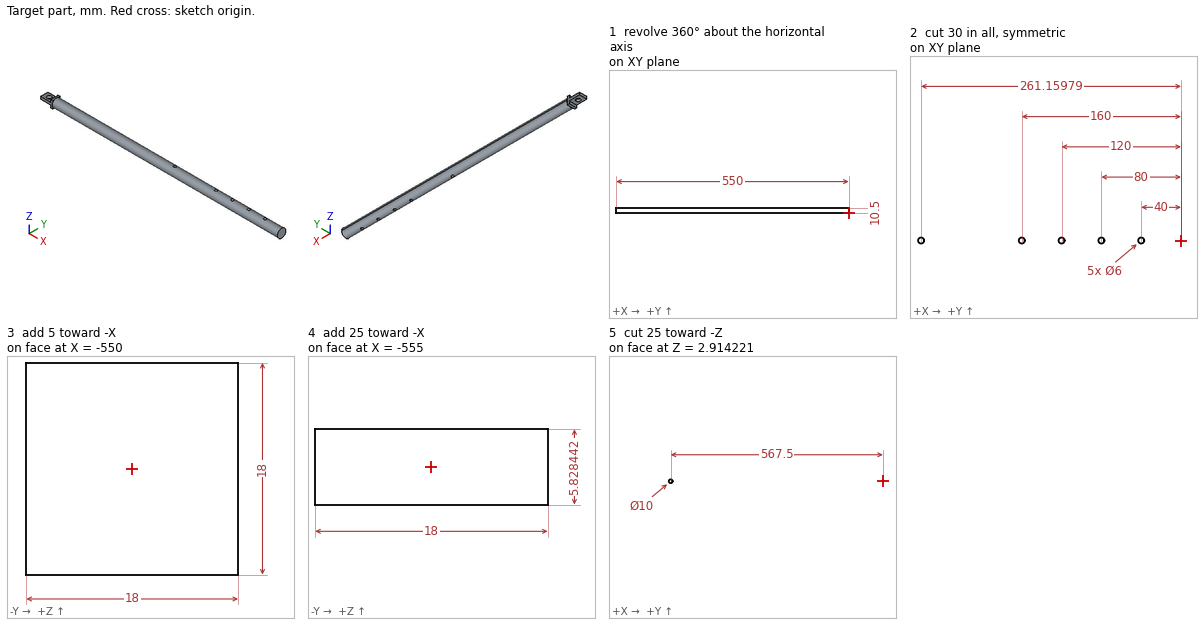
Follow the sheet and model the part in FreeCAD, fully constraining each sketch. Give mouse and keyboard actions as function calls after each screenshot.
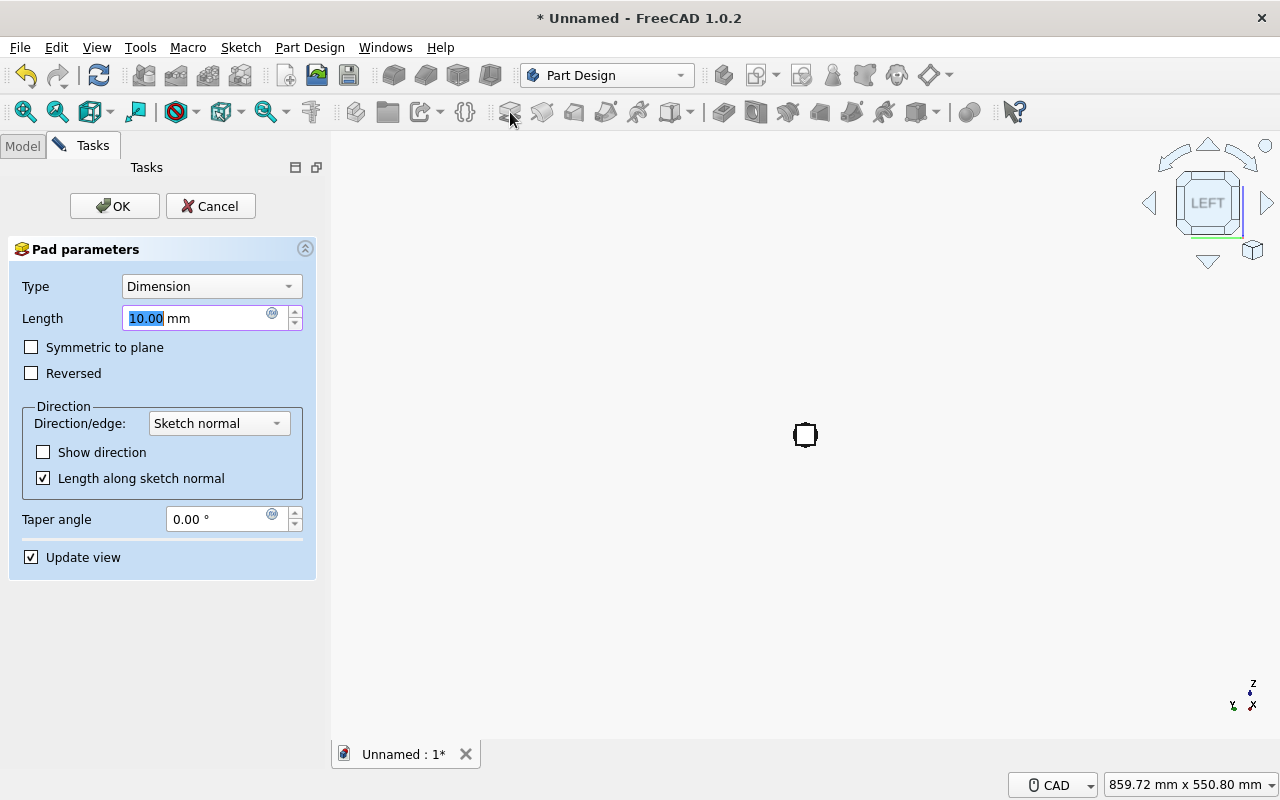
text(5)
key(Tab)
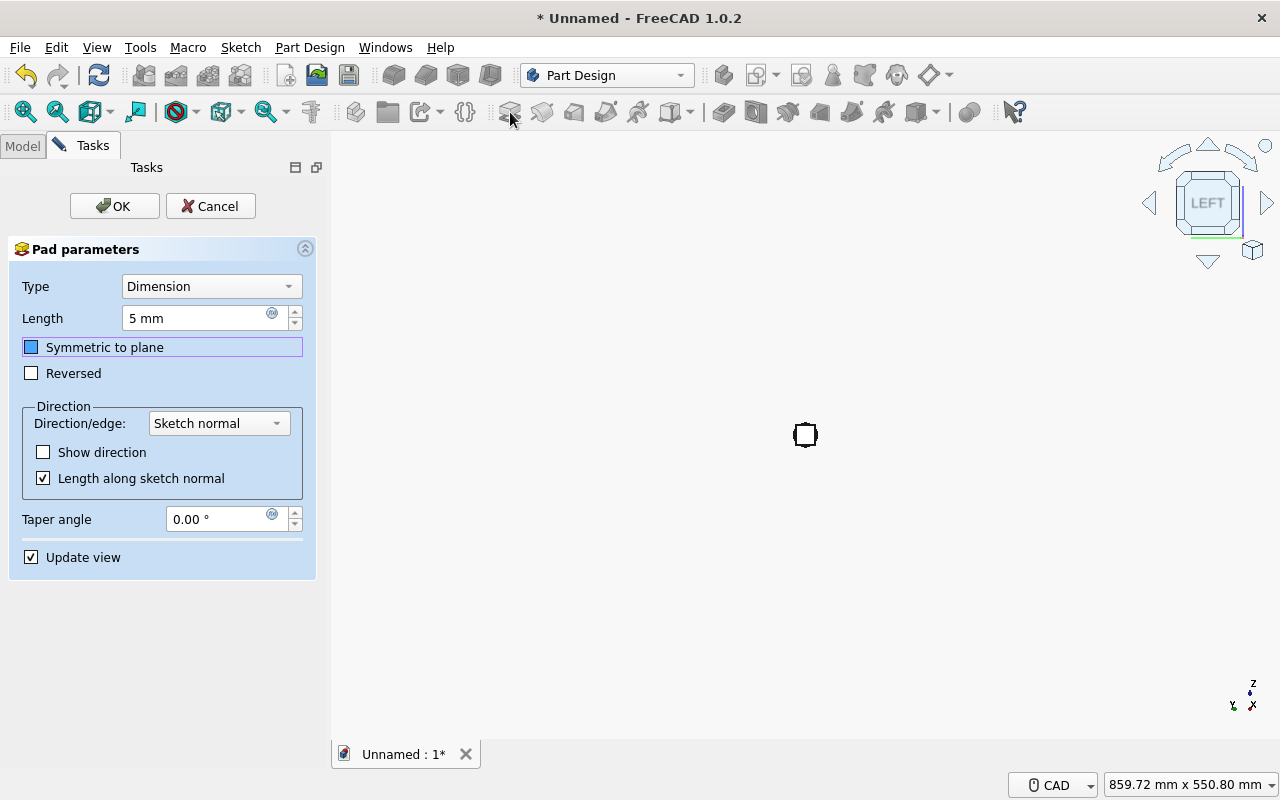
click(115, 206)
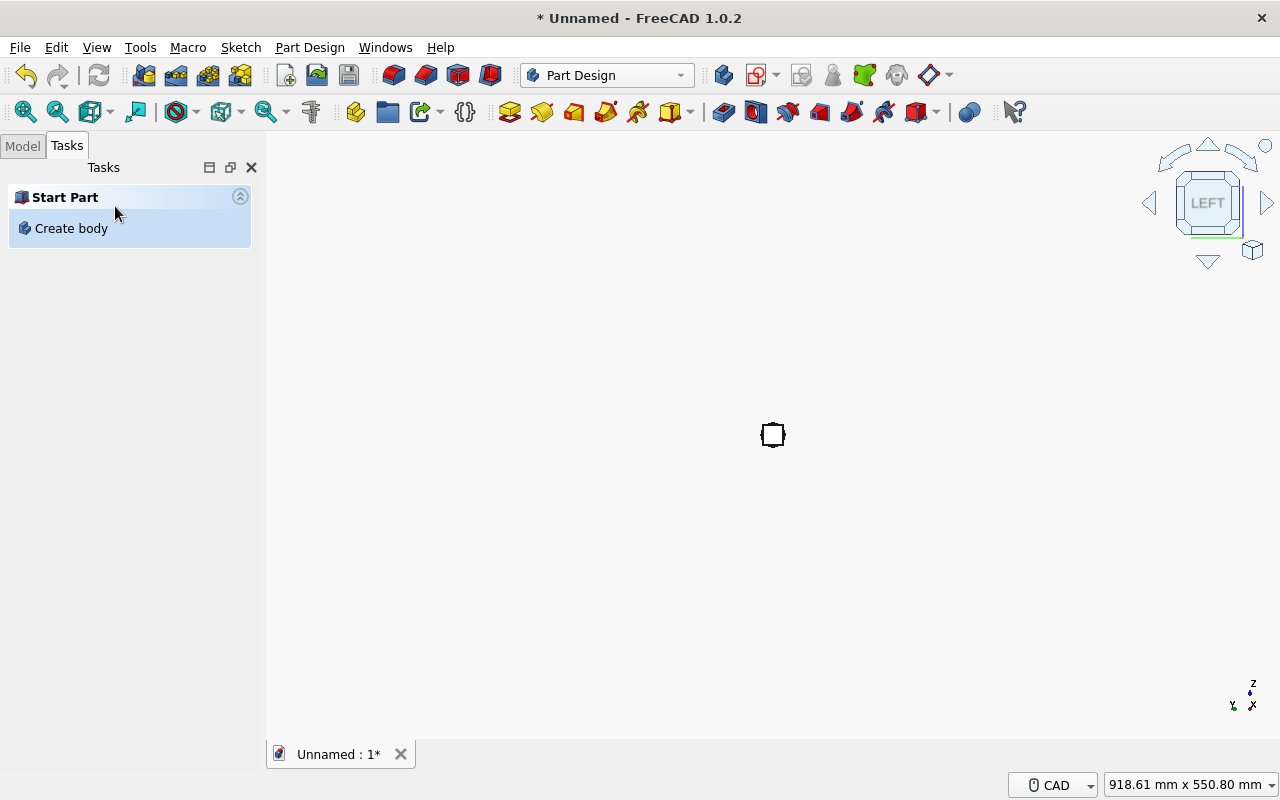
key(v)
key(f)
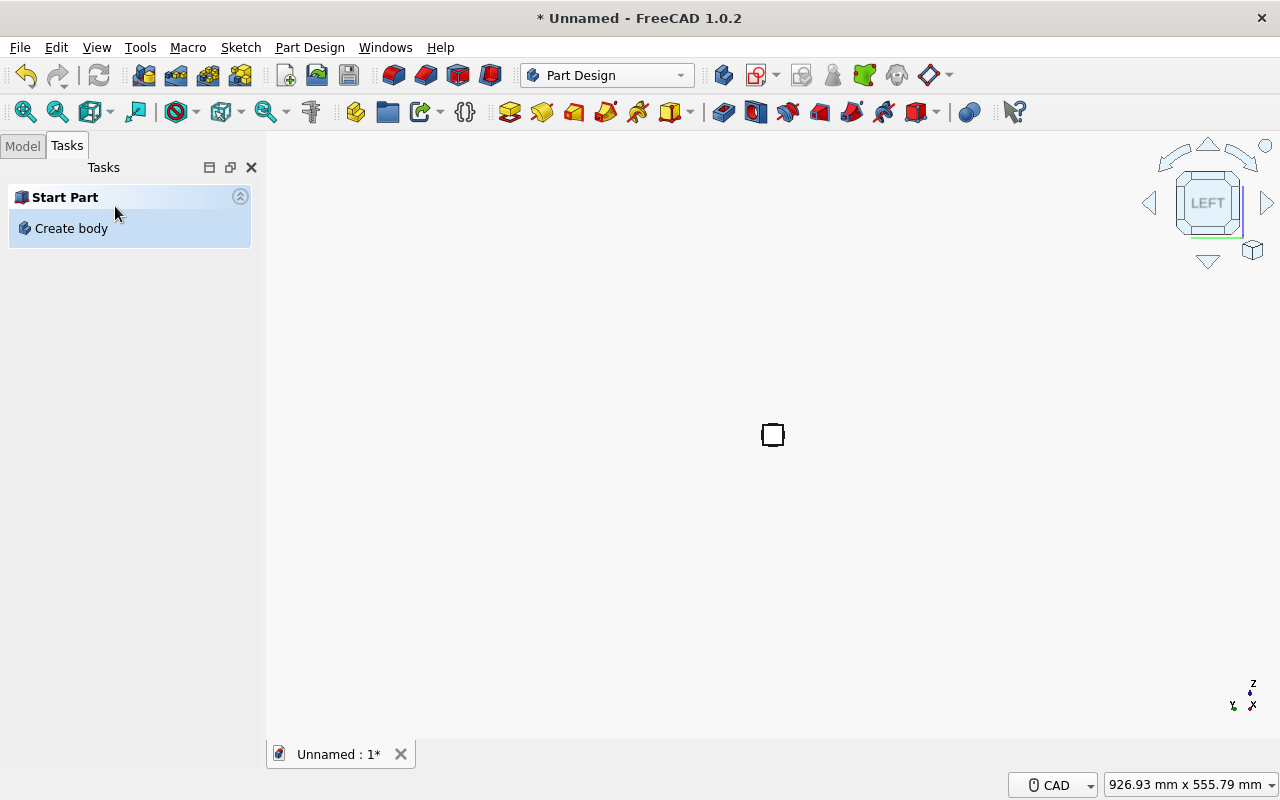
click(773, 434)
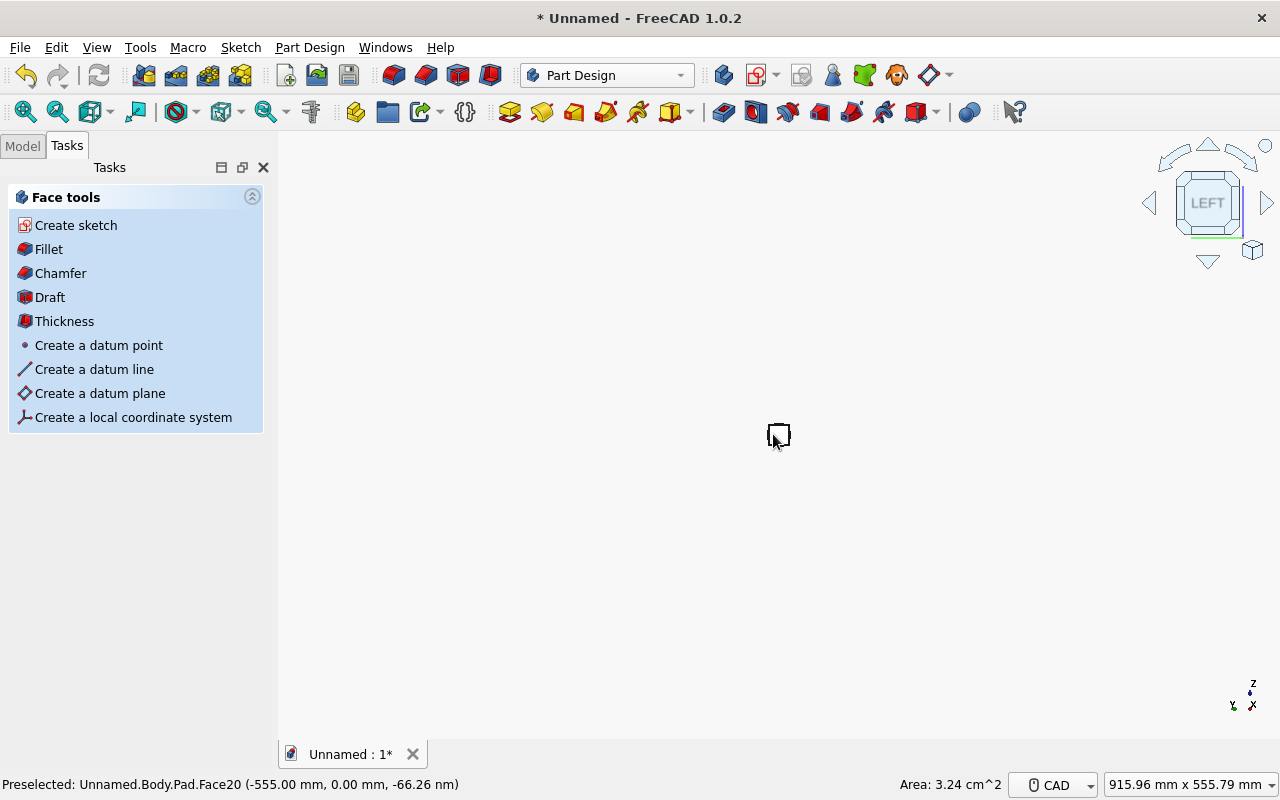
click(756, 76)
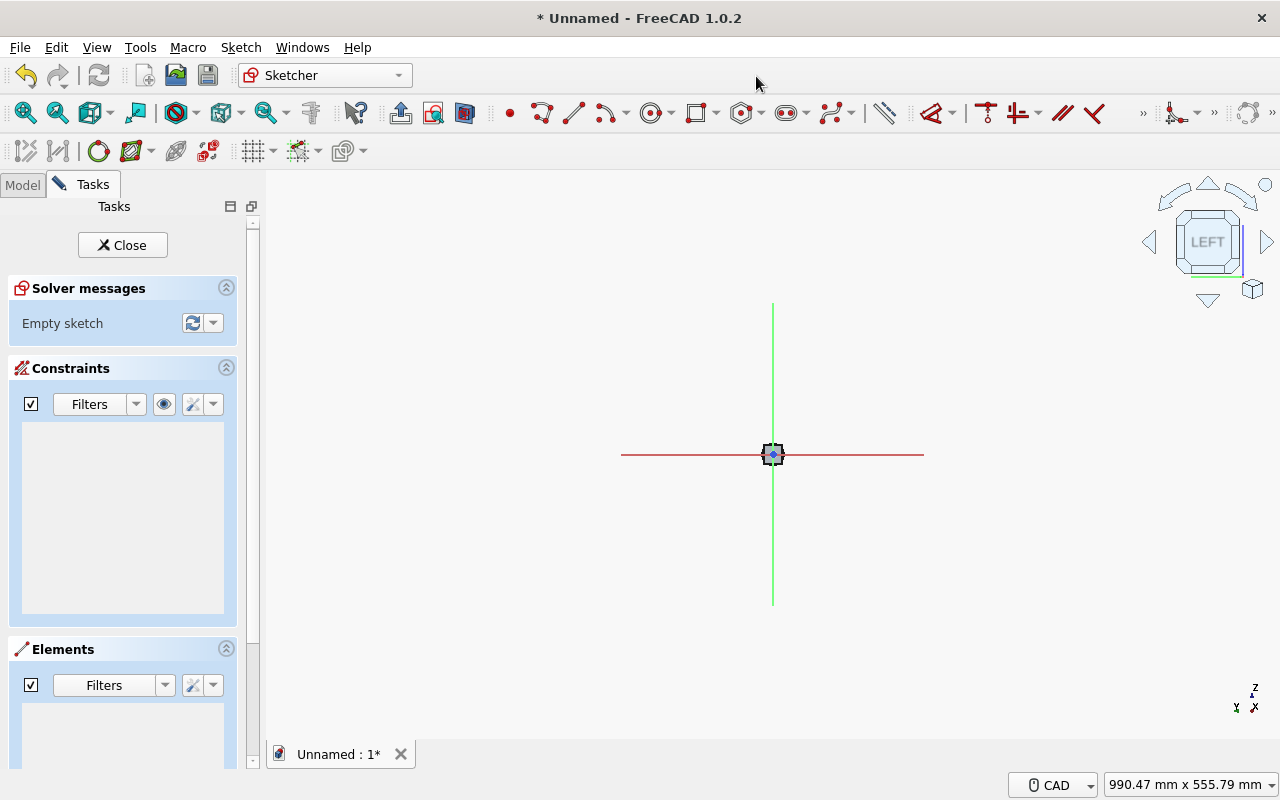
scroll(777, 455, up, 15)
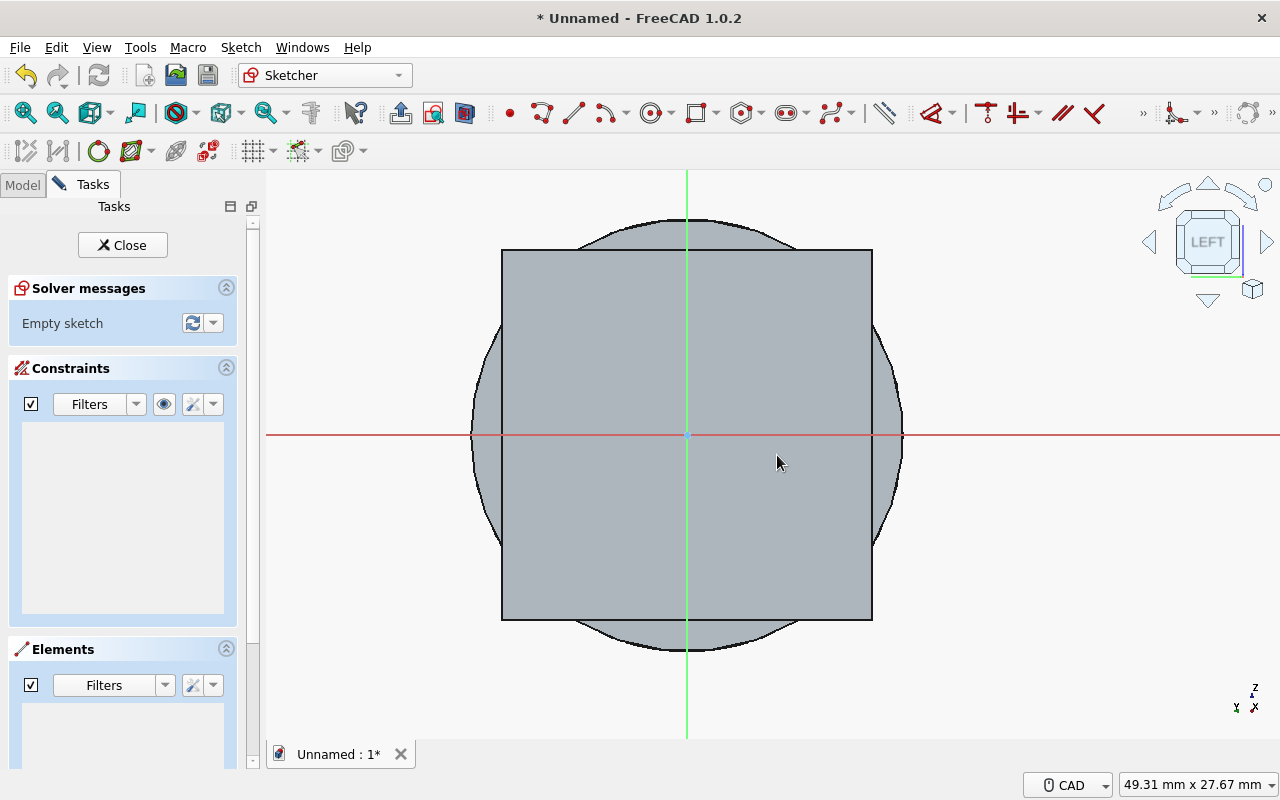
scroll(652, 397, up, 2)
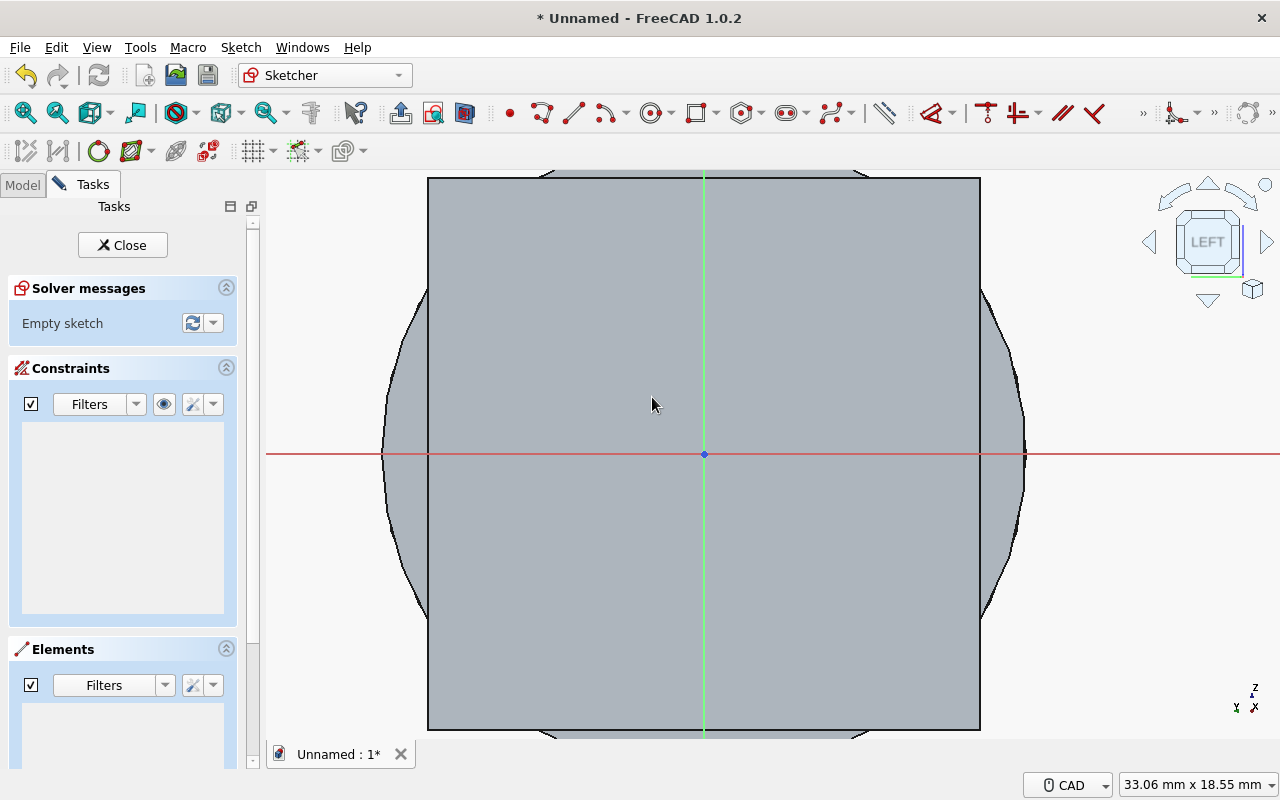
key(g)
key(v)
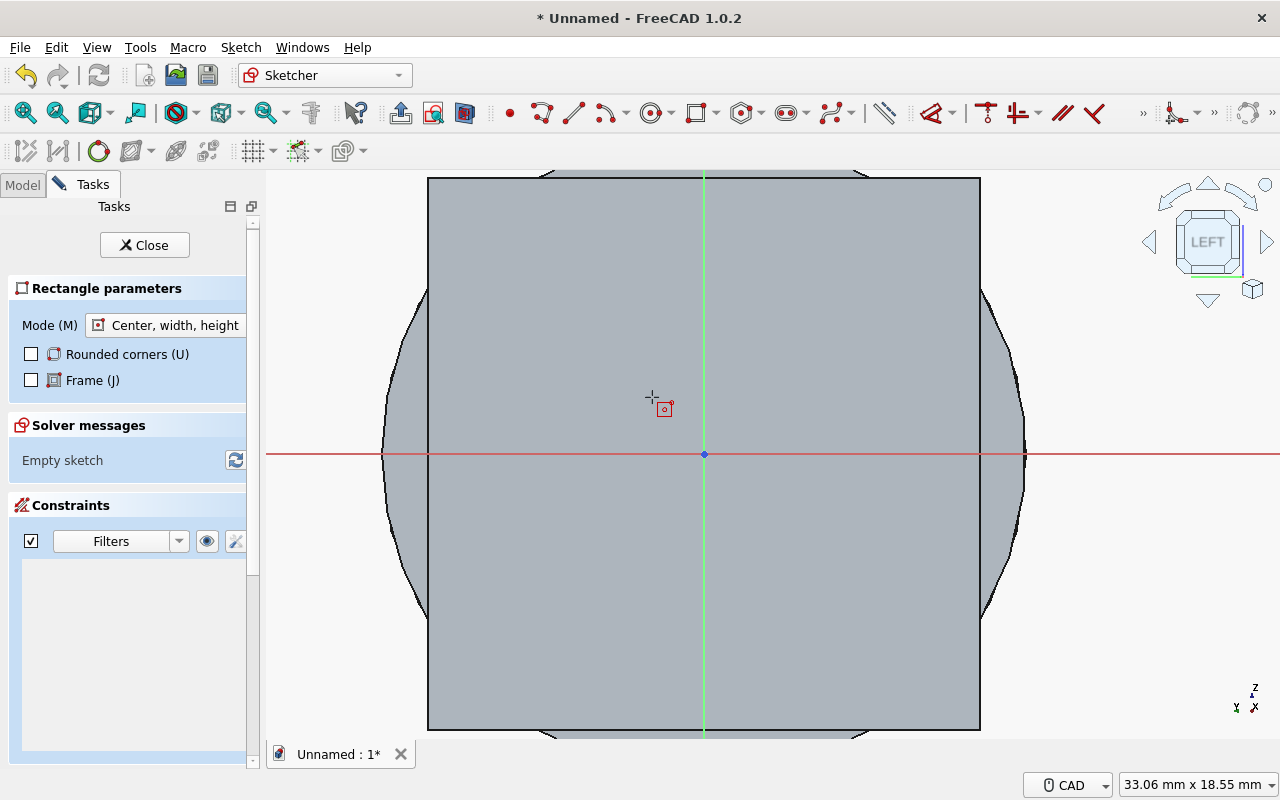
click(704, 454)
click(980, 365)
key(Escape)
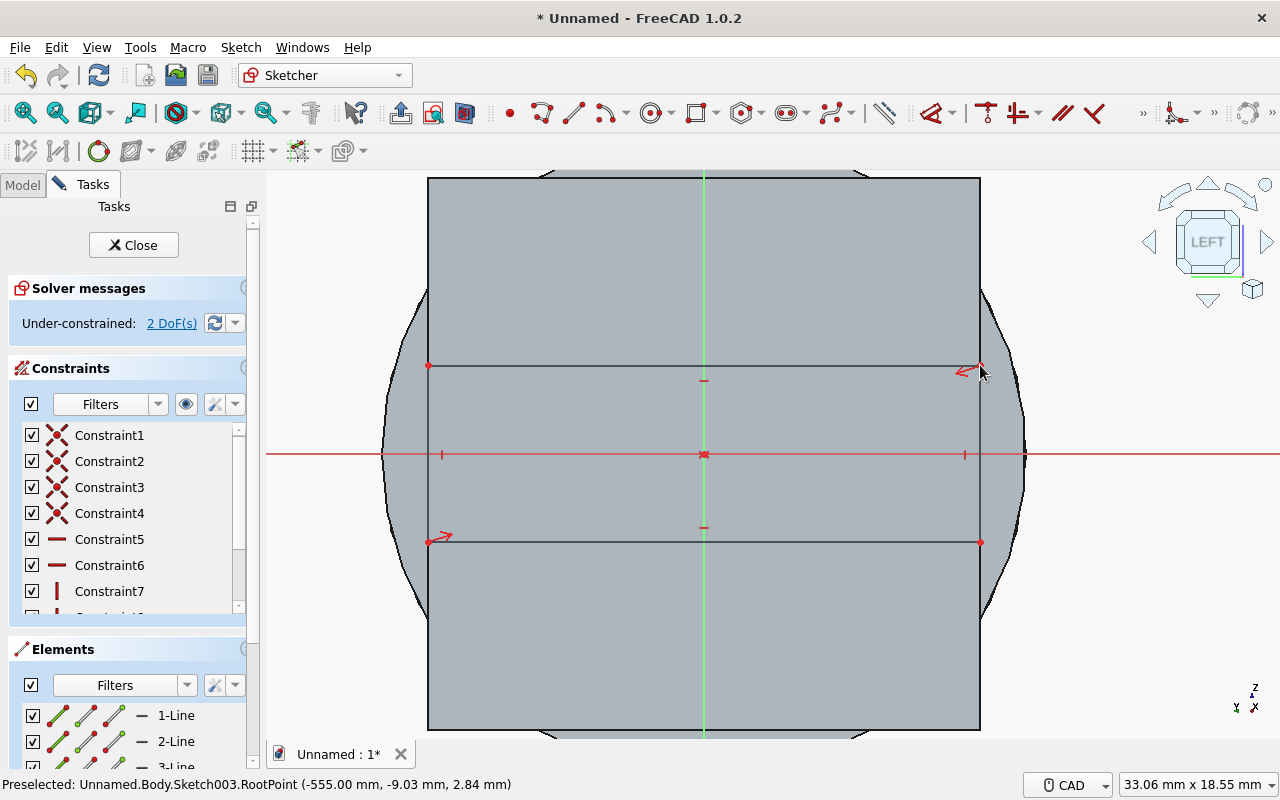
key(d)